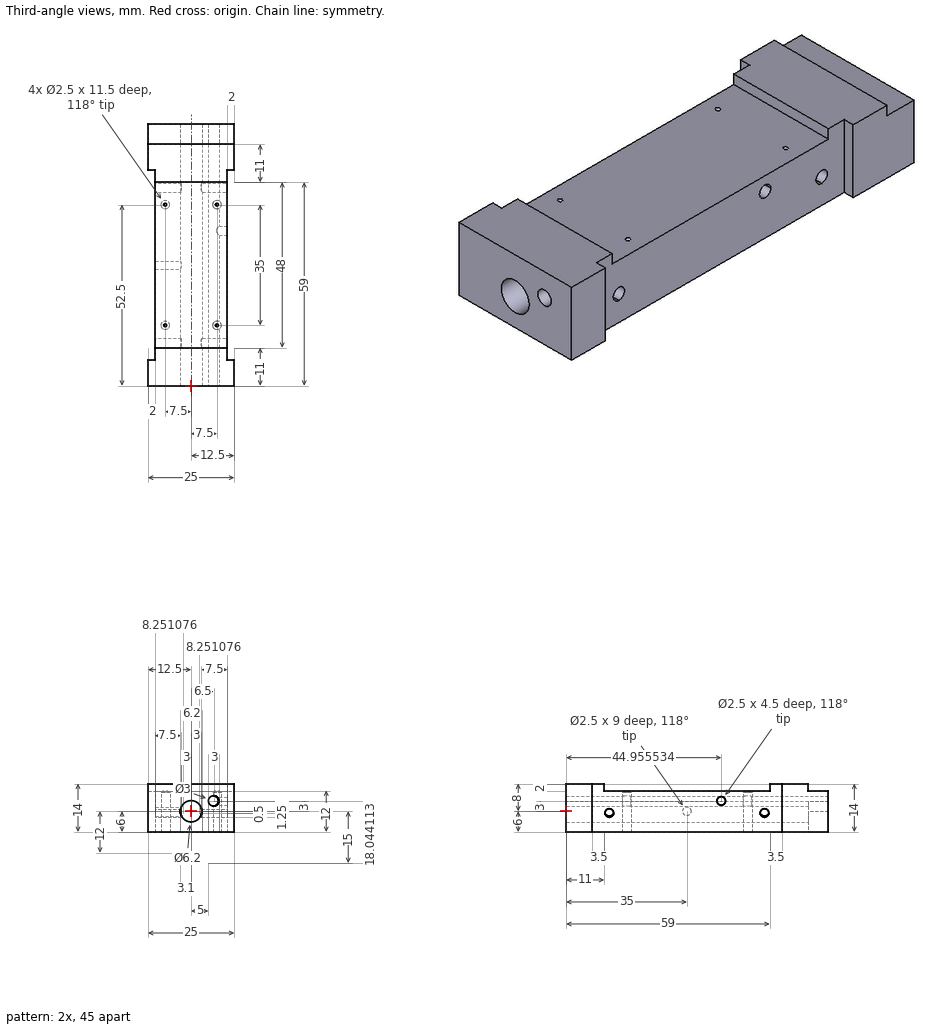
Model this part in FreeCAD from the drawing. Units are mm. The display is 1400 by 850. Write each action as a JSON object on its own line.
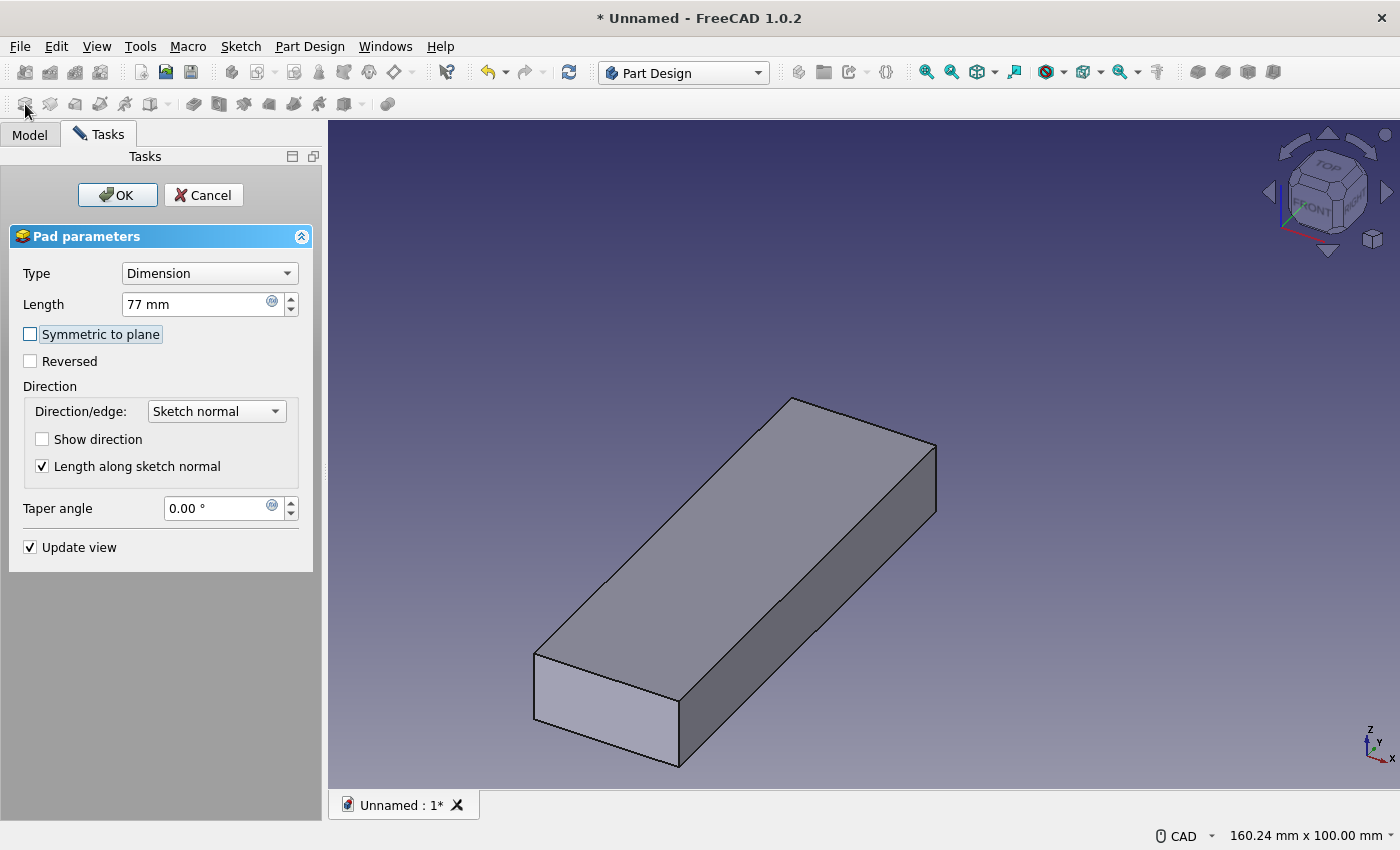
{"action": "left_click", "coordinate": [31, 361]}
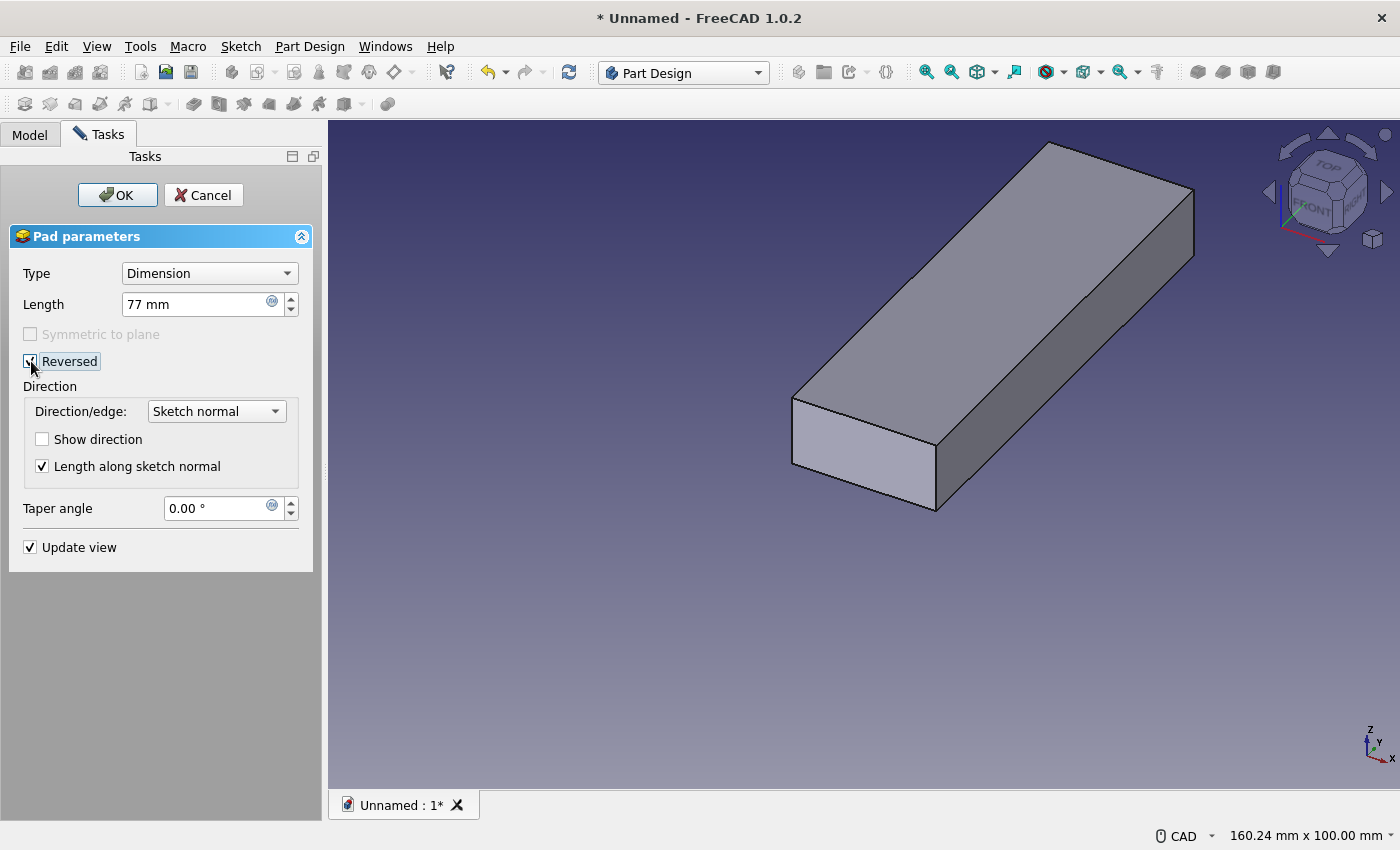
{"action": "left_click", "coordinate": [118, 195]}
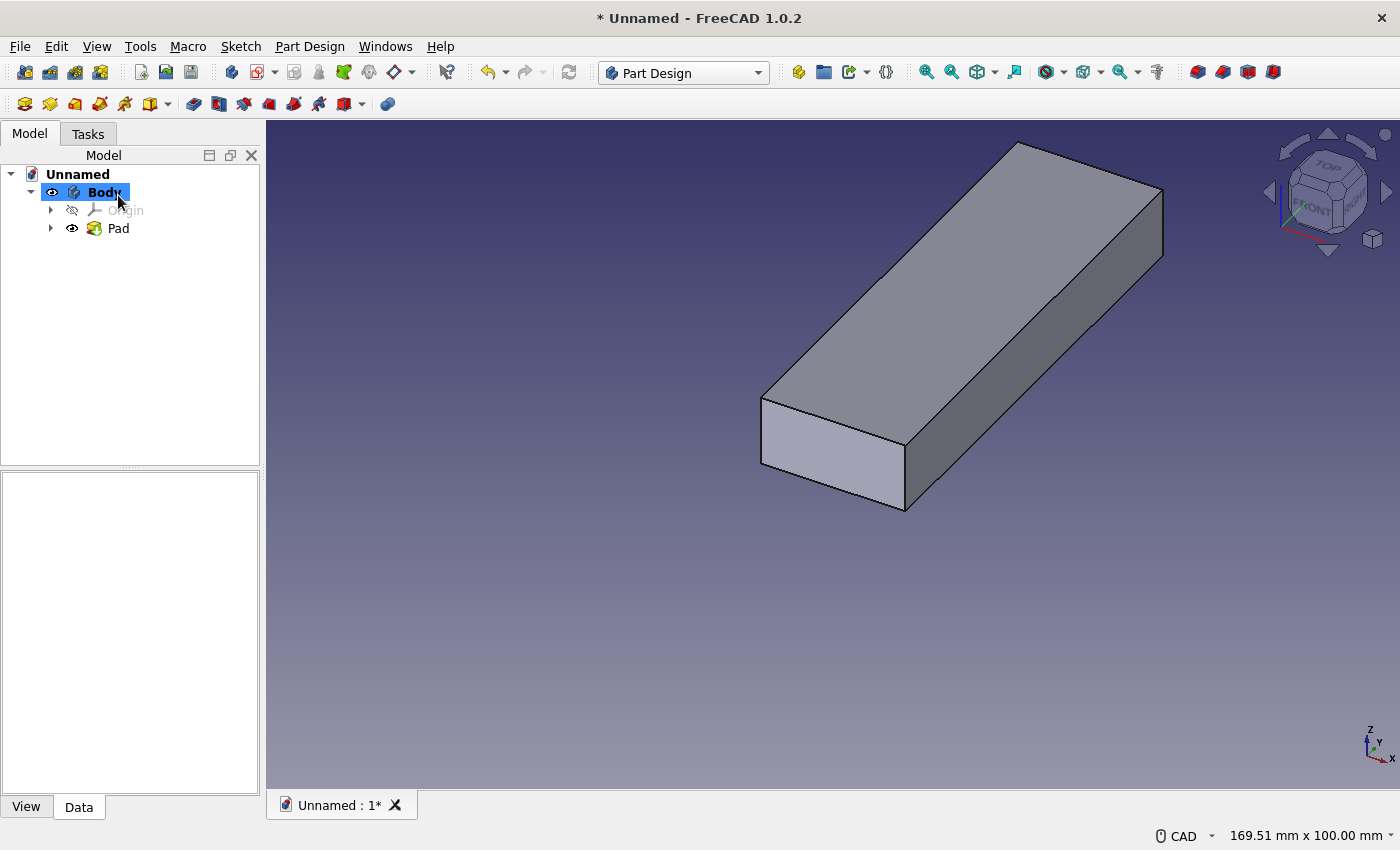
{"action": "left_click", "coordinate": [256, 72]}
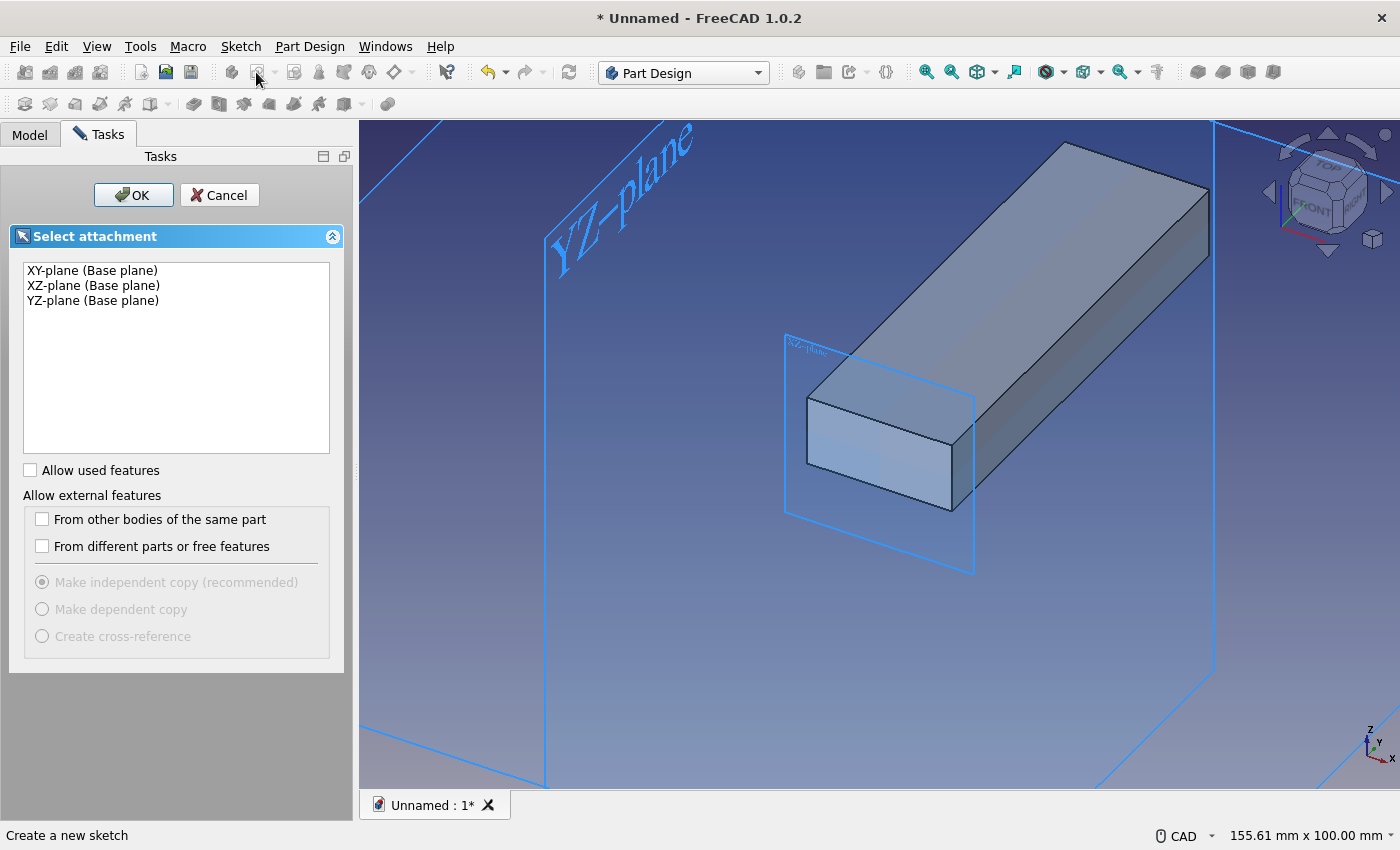
{"action": "left_click", "coordinate": [84, 286]}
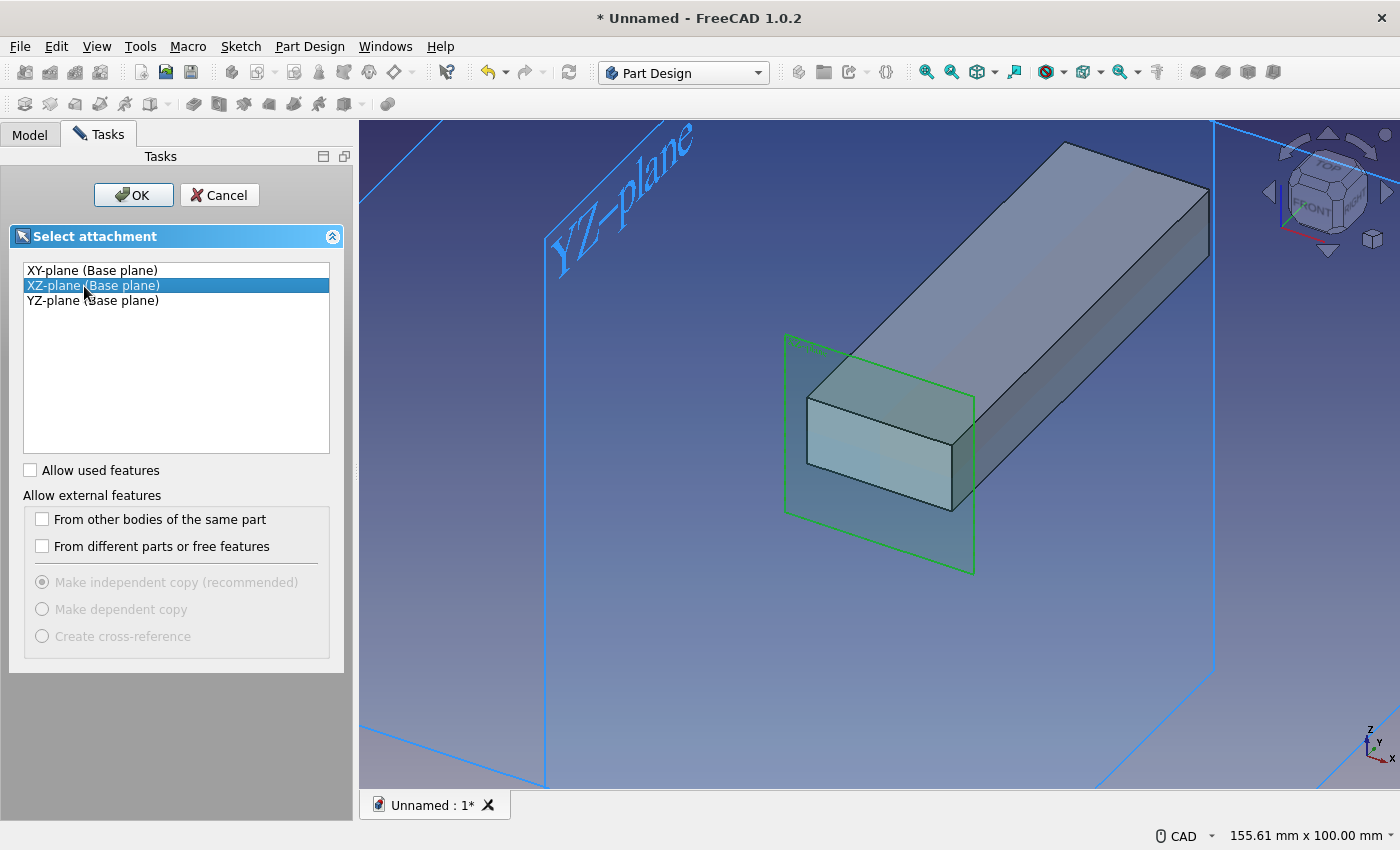
{"action": "left_click", "coordinate": [134, 195]}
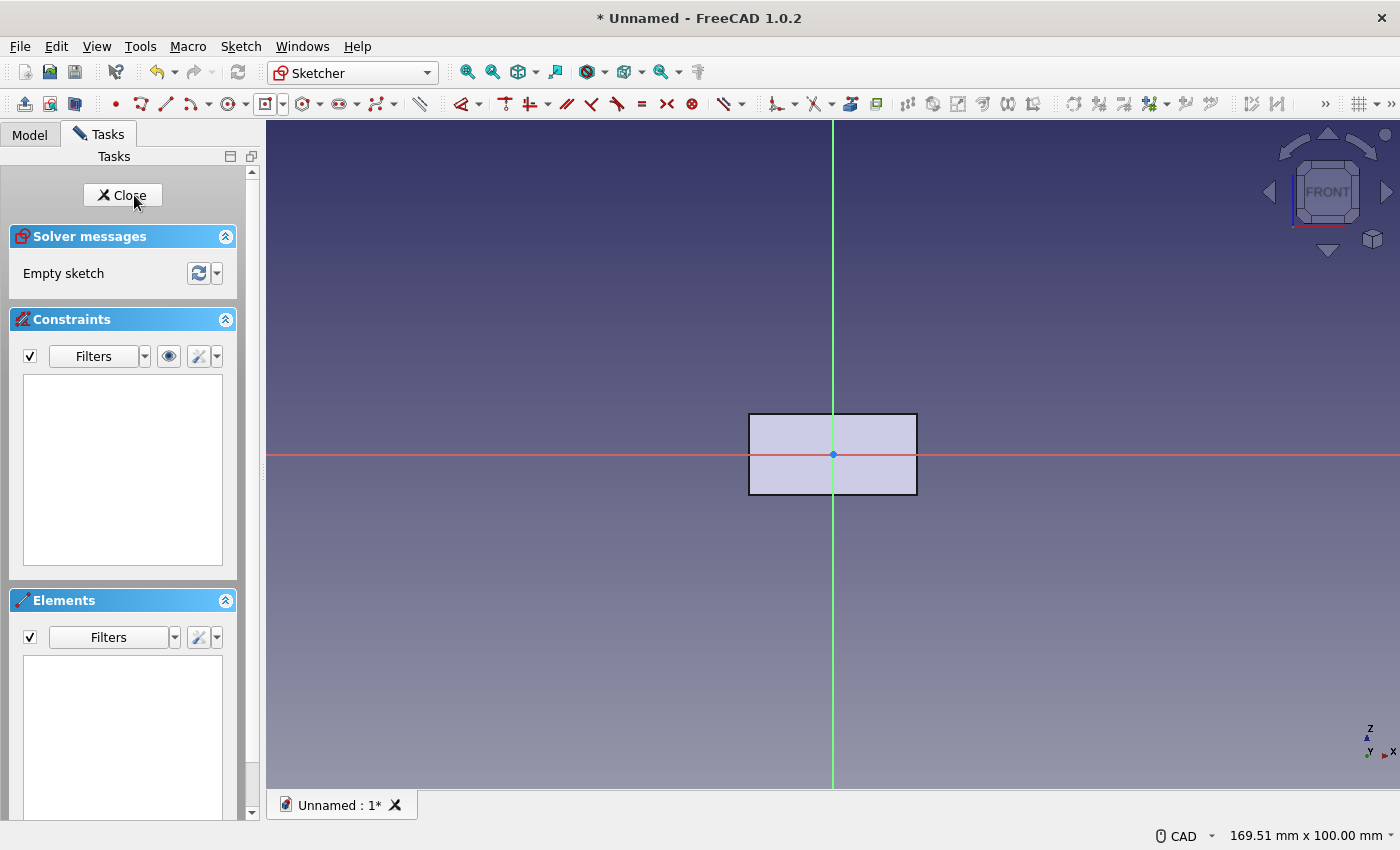
{"action": "scroll", "coordinate": [860, 449], "scroll_direction": "up", "scroll_amount": 11}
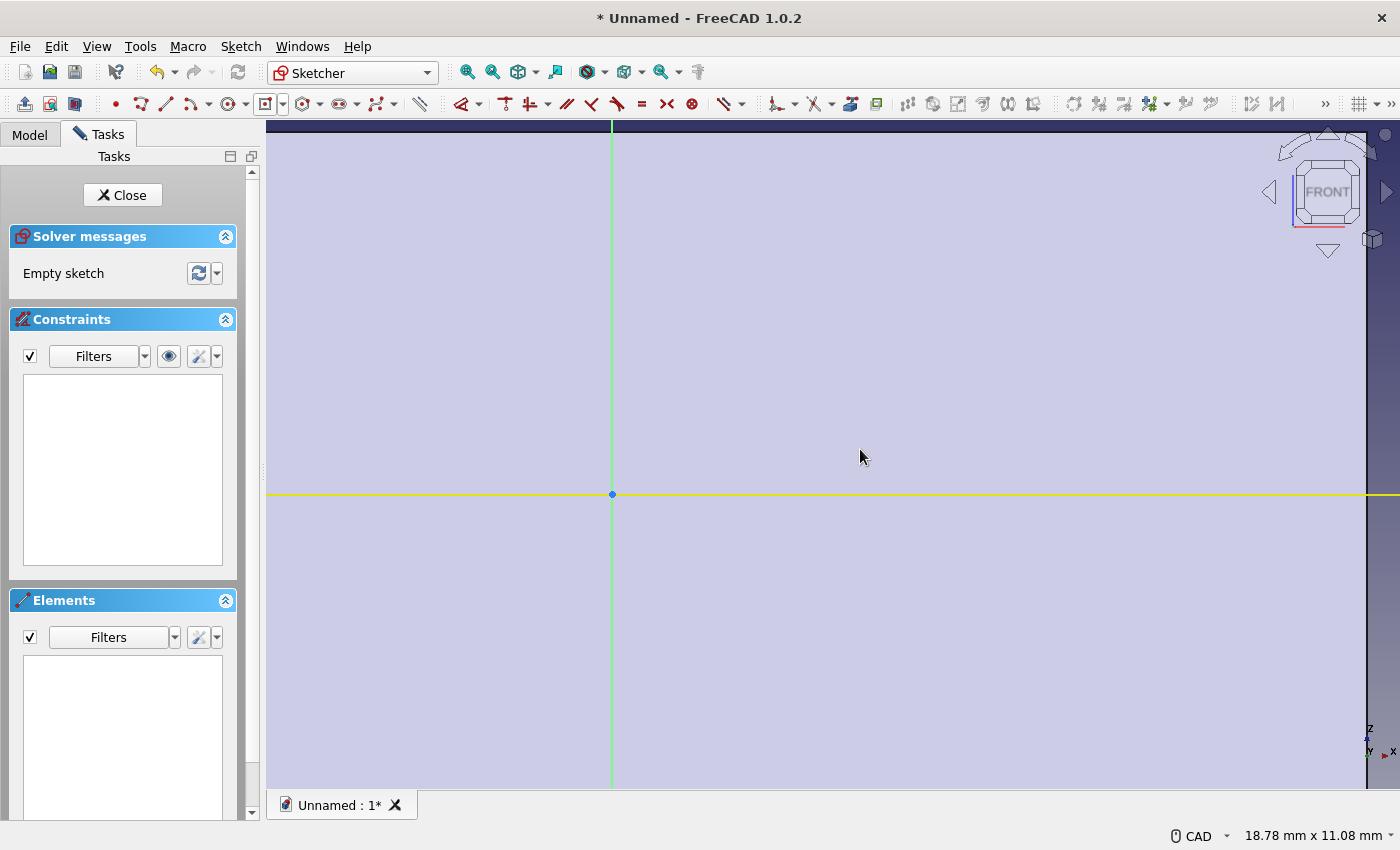
{"action": "left_click", "coordinate": [228, 104]}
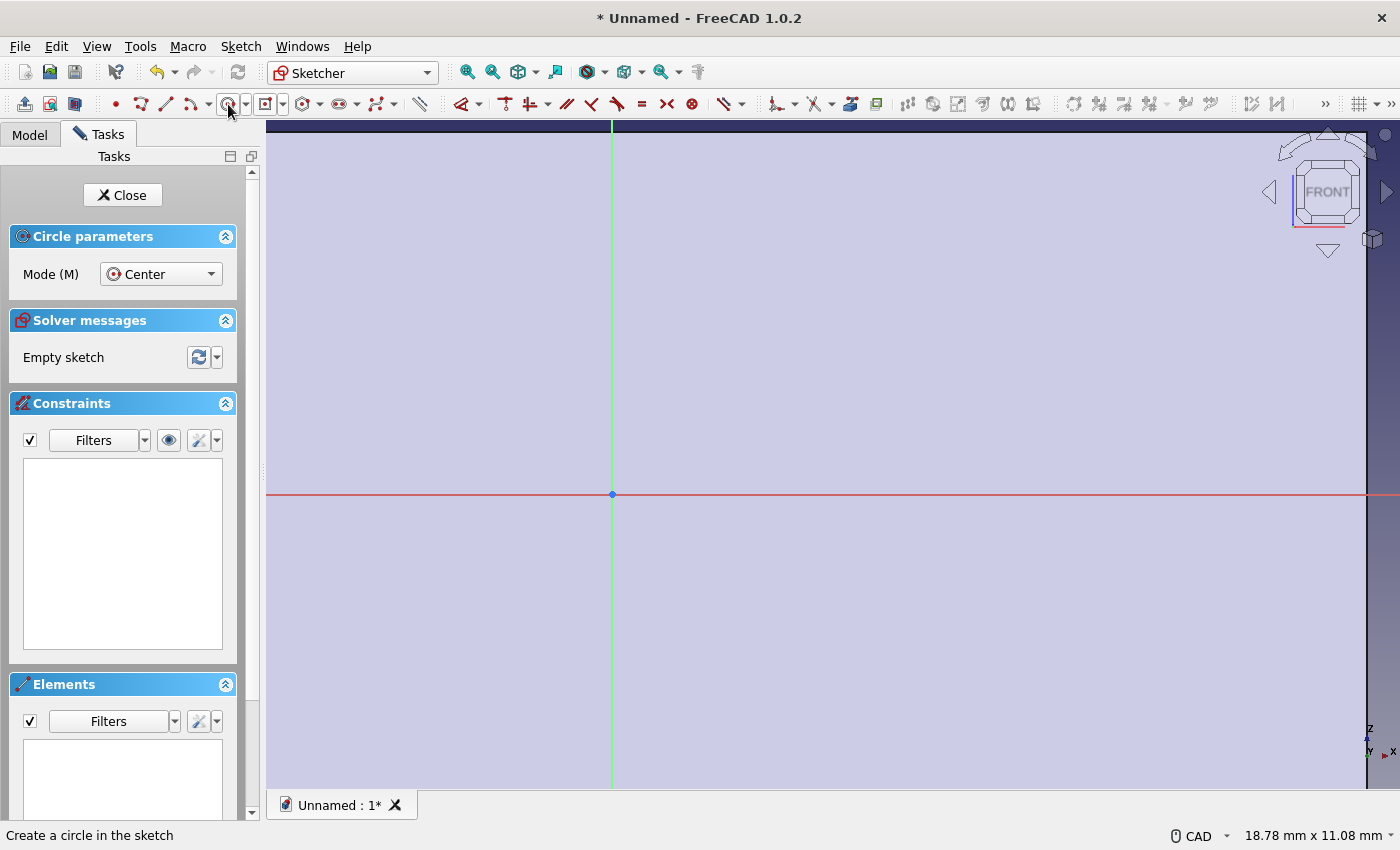
{"action": "left_click", "coordinate": [612, 495]}
{"action": "left_click", "coordinate": [744, 362]}